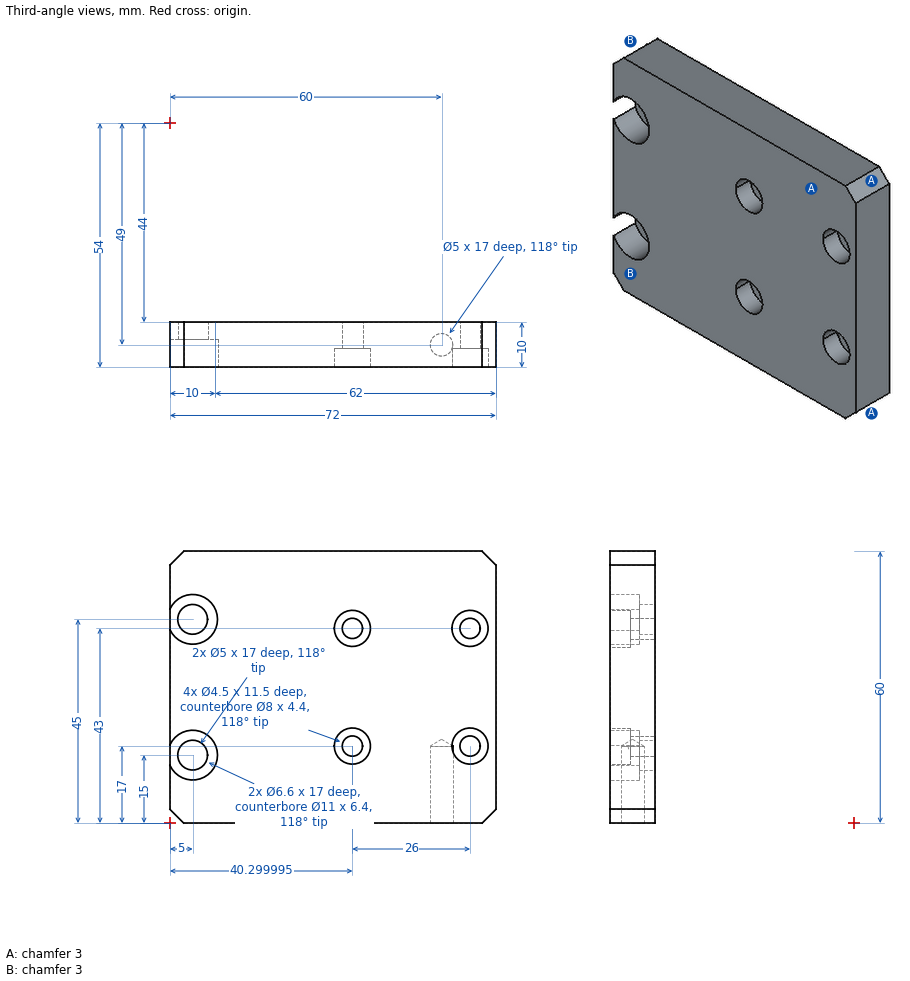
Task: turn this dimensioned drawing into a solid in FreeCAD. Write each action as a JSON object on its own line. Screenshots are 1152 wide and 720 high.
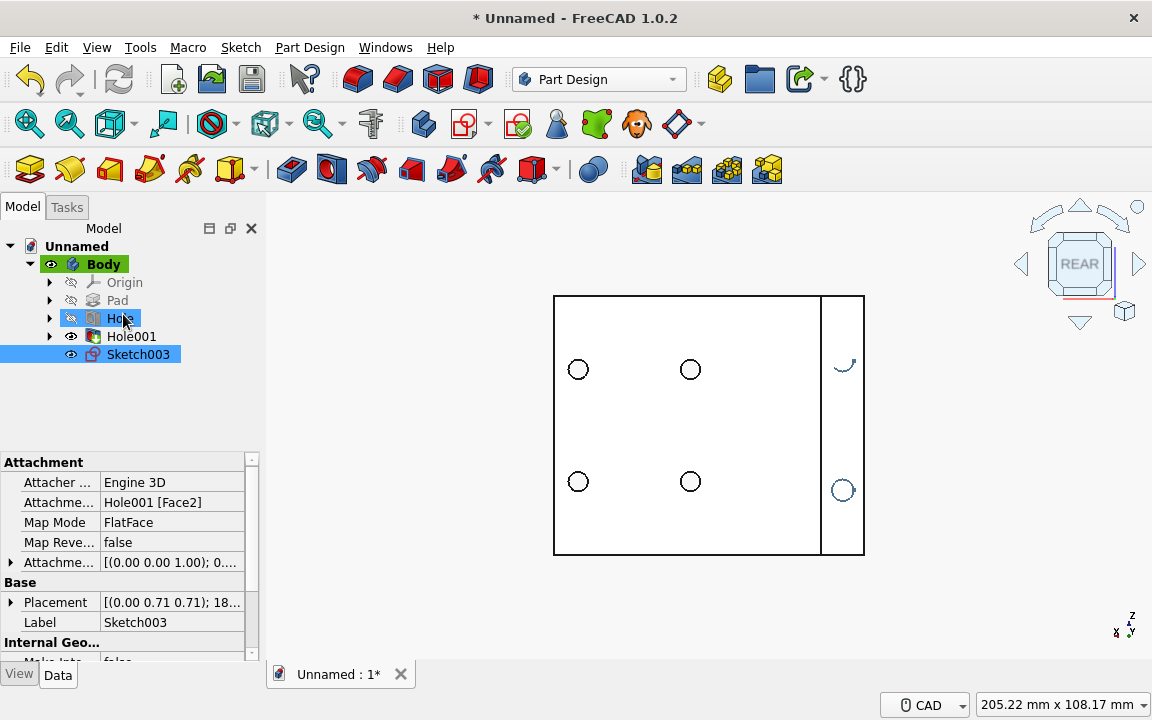
{"action": "left_click", "coordinate": [332, 170]}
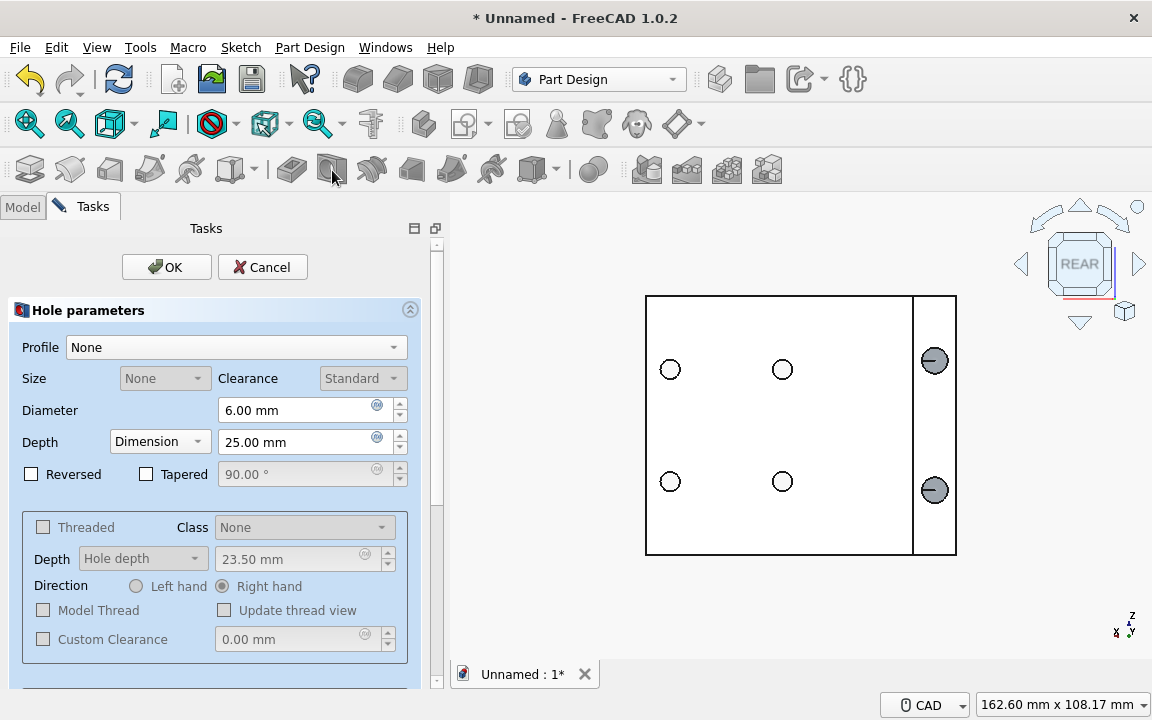
{"action": "triple_click", "coordinate": [305, 410]}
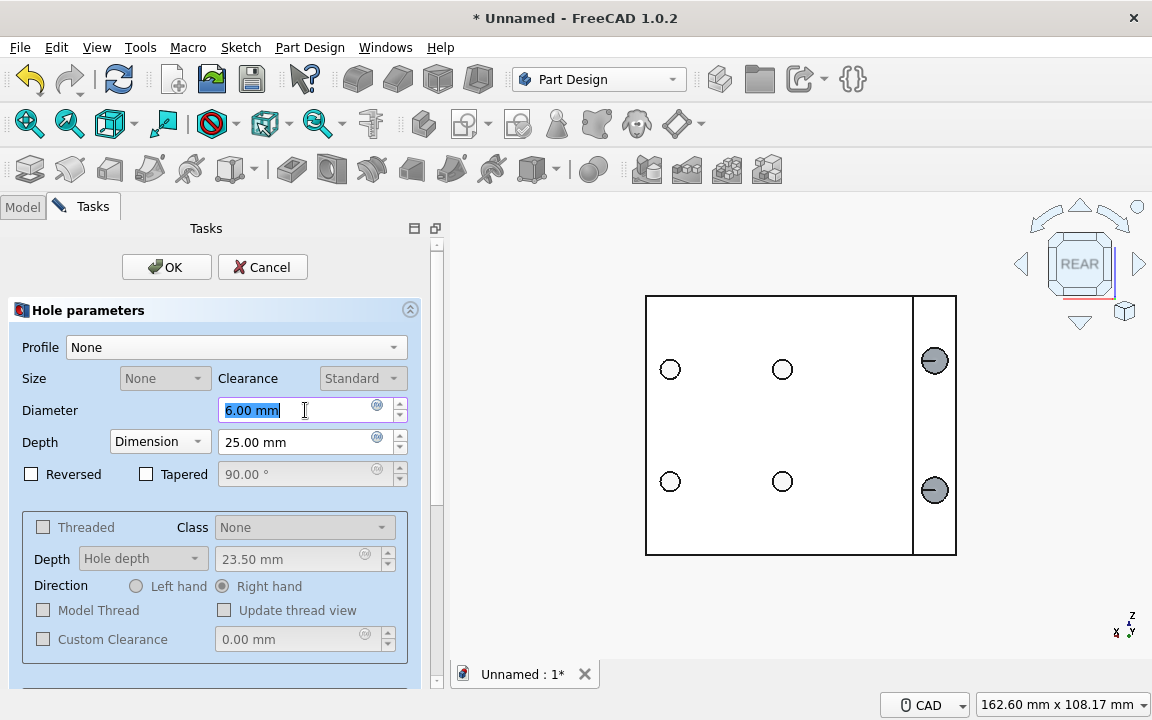
{"action": "type", "text": "5"}
{"action": "key", "text": "Tab"}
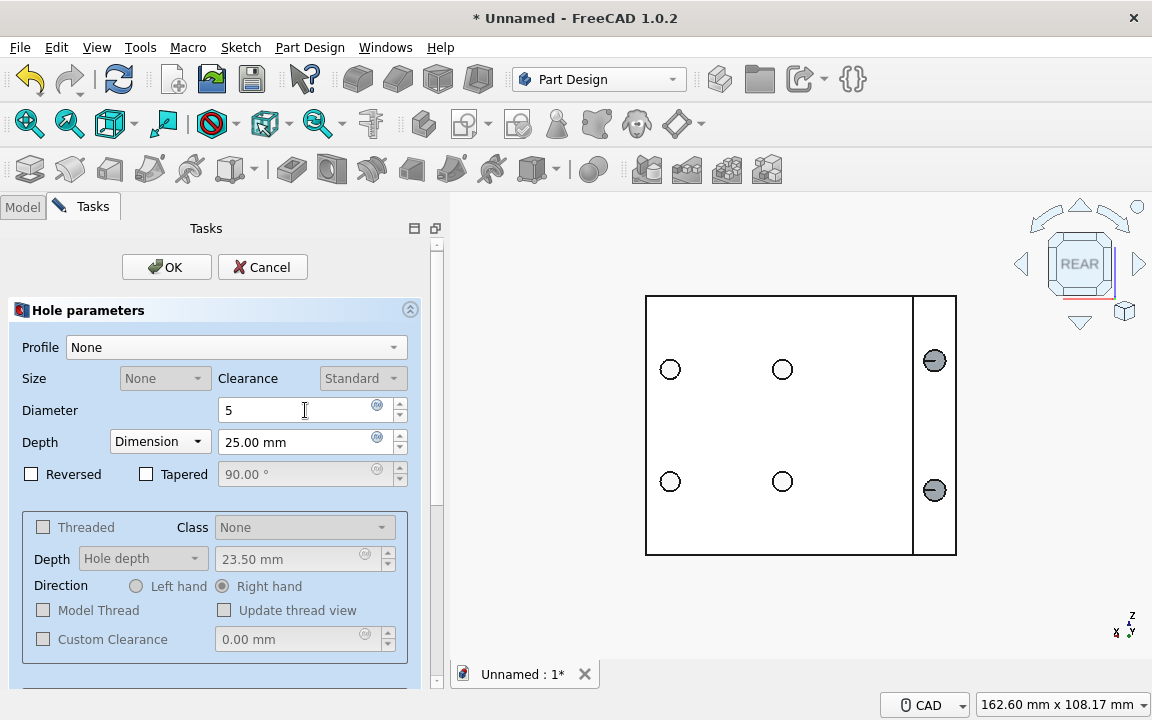
{"action": "triple_click", "coordinate": [305, 442]}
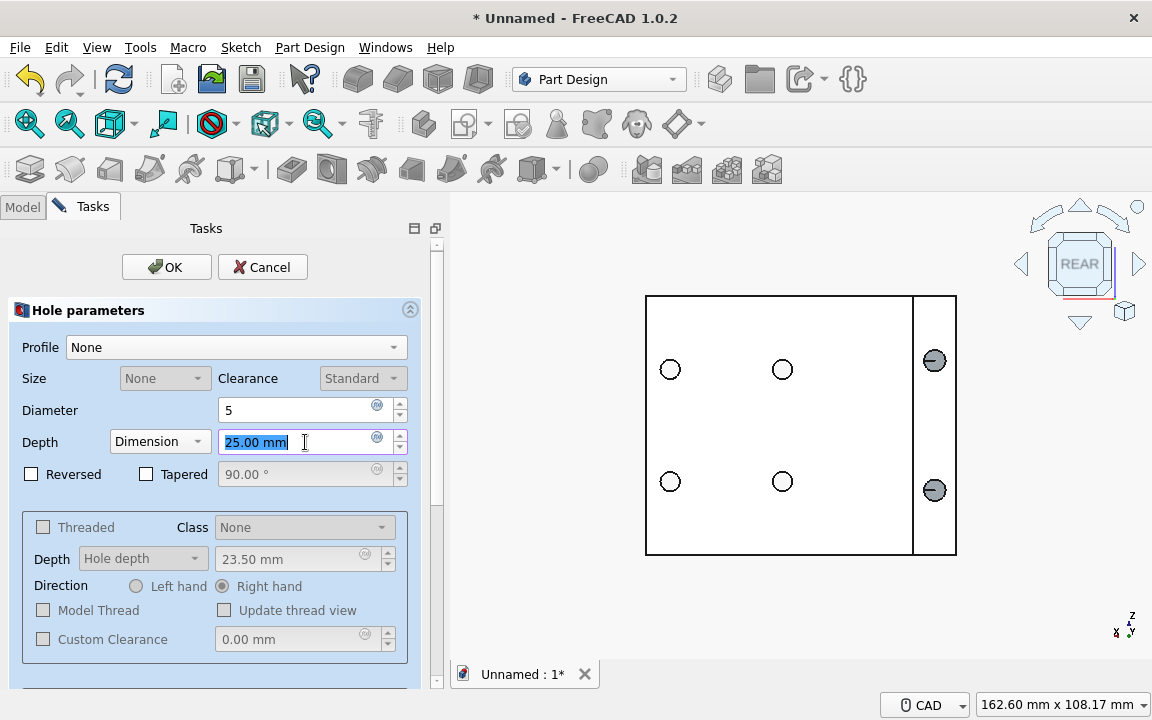
{"action": "type", "text": "17"}
{"action": "key", "text": "Tab"}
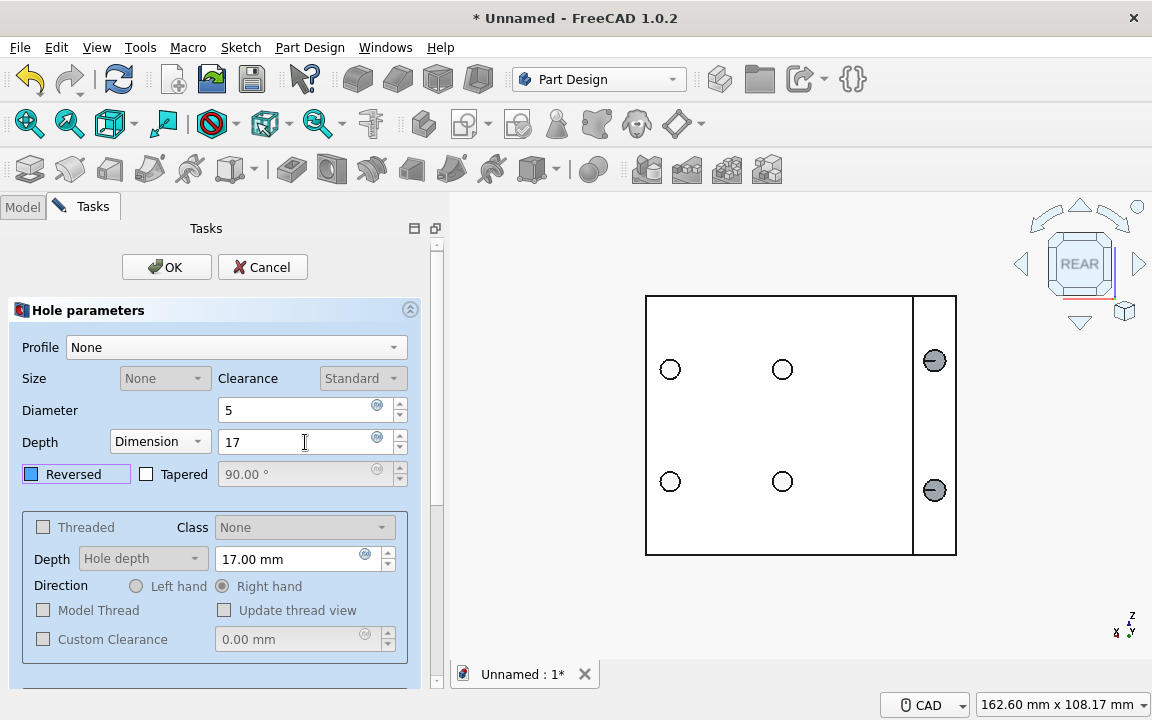
{"action": "left_click", "coordinate": [167, 267]}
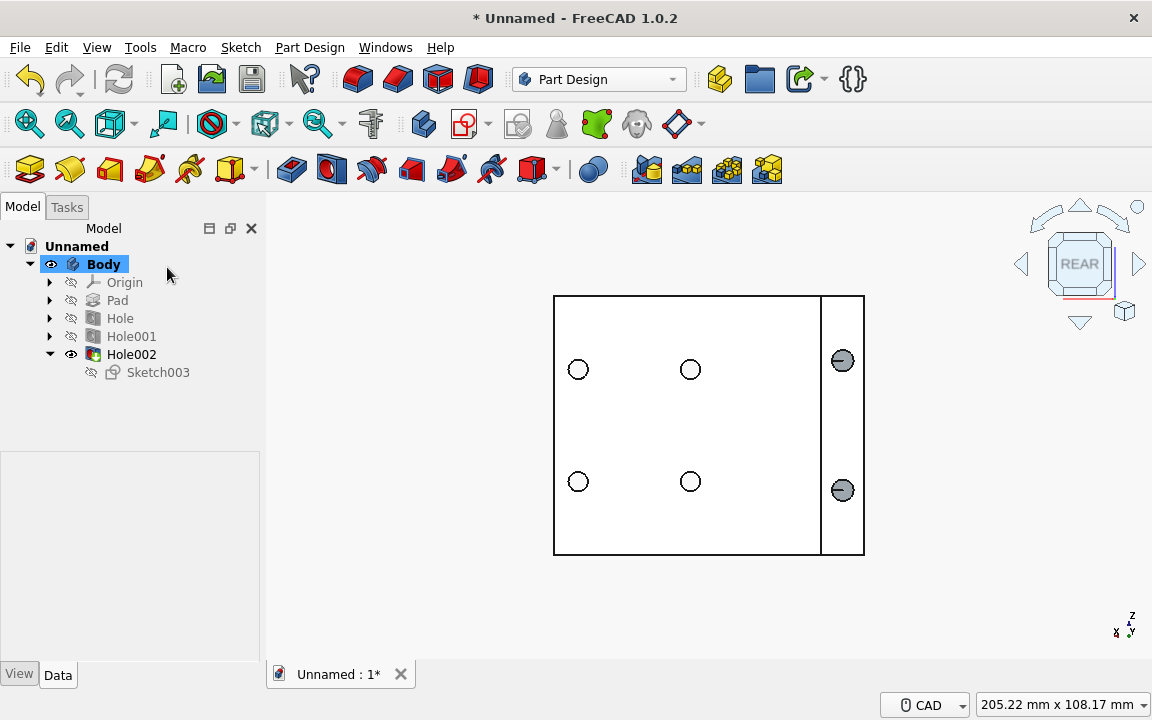
{"action": "left_click", "coordinate": [843, 295]}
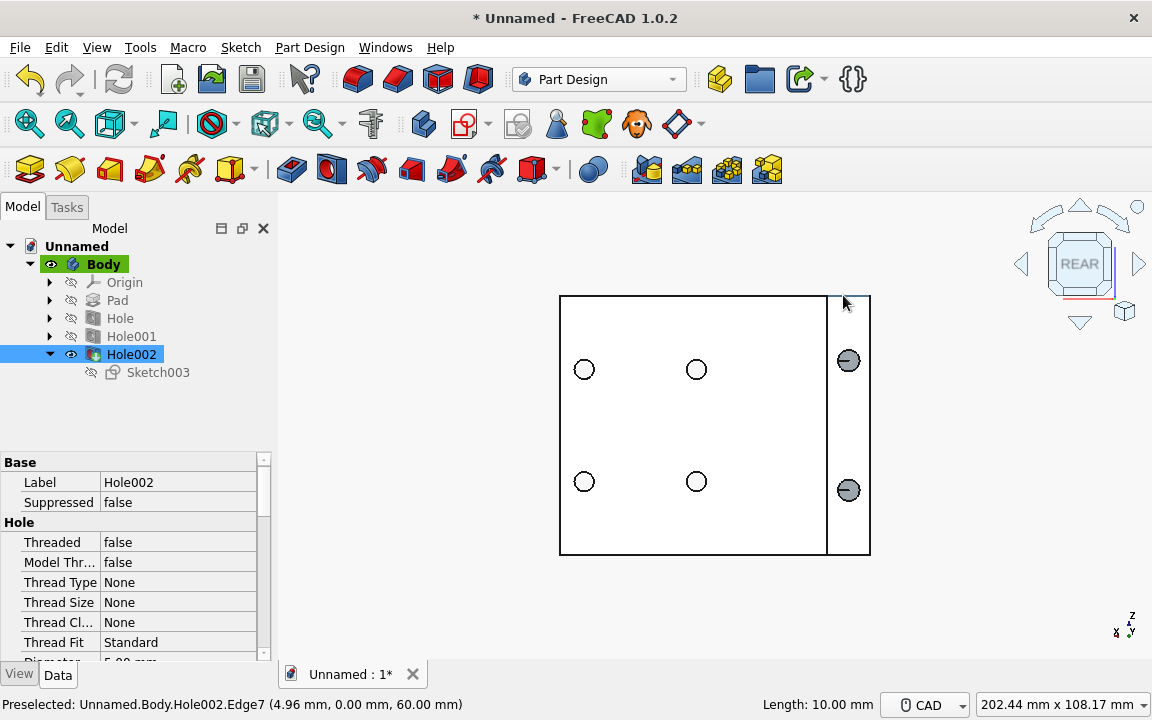
{"action": "key", "text": "0"}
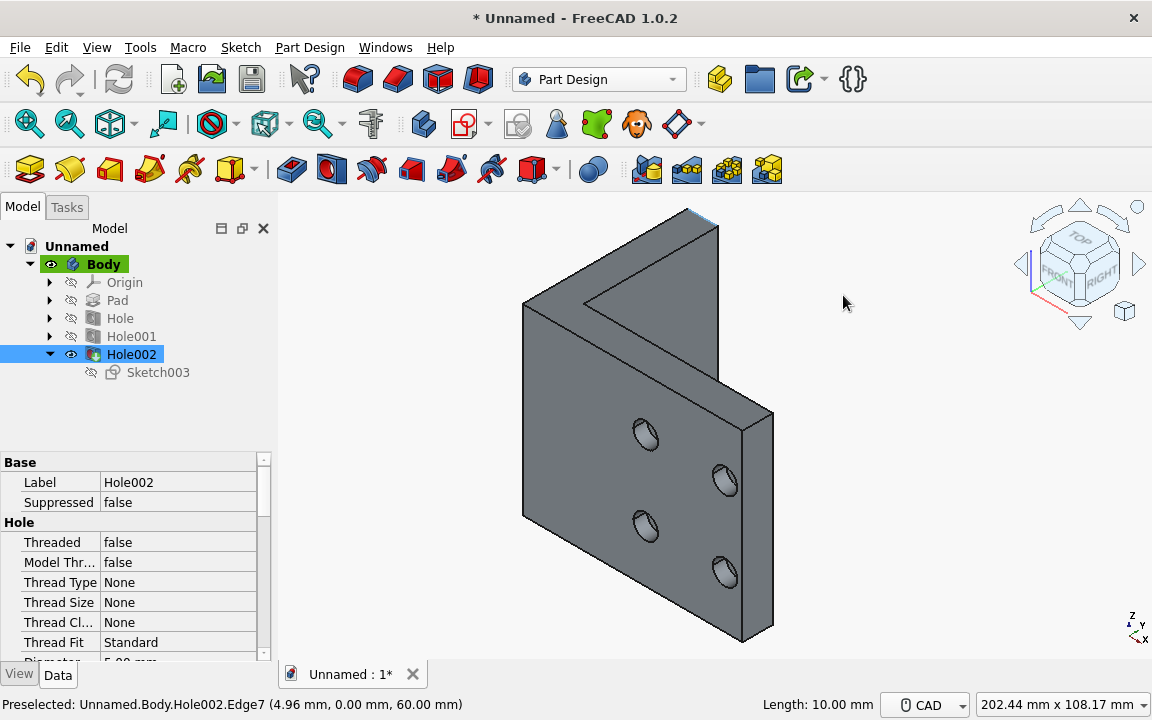
{"action": "left_click", "coordinate": [758, 421], "text": "ctrl"}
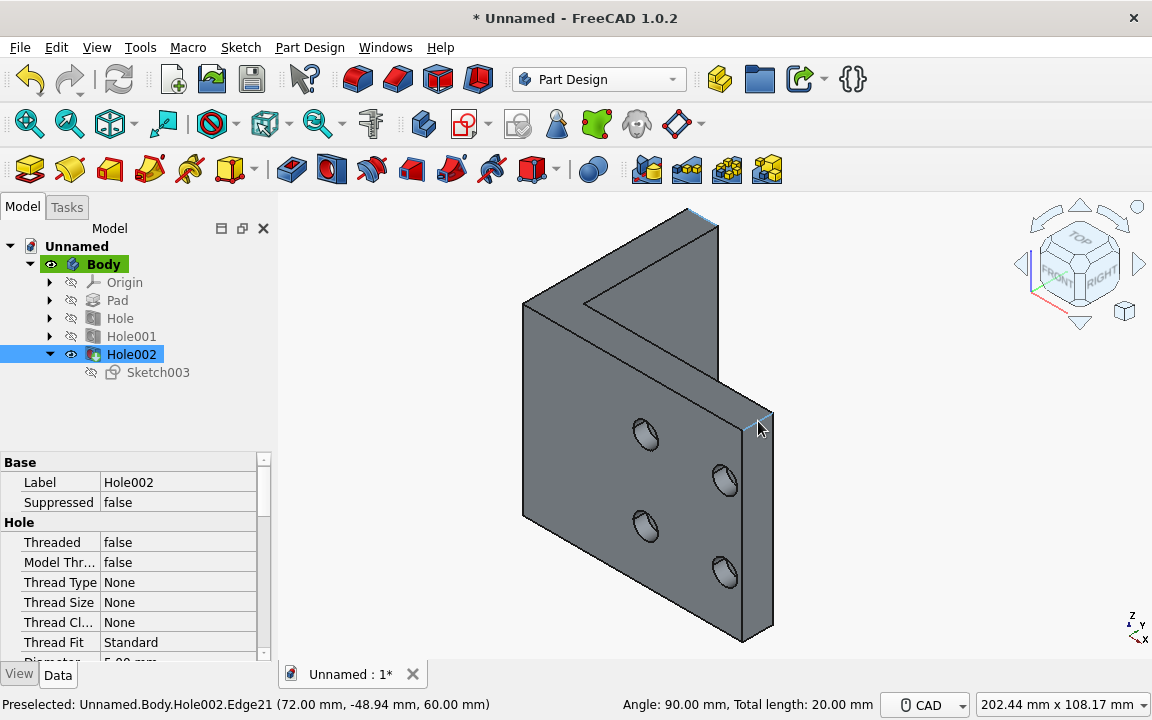
{"action": "key", "text": "2"}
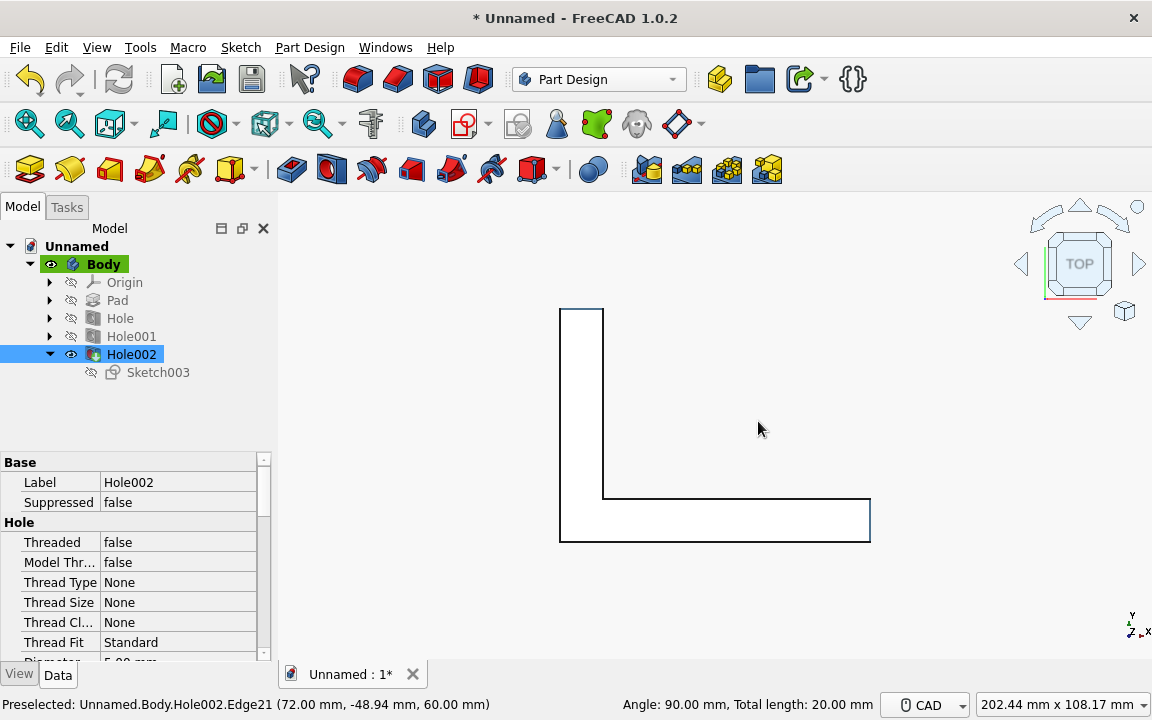
{"action": "key", "text": "1"}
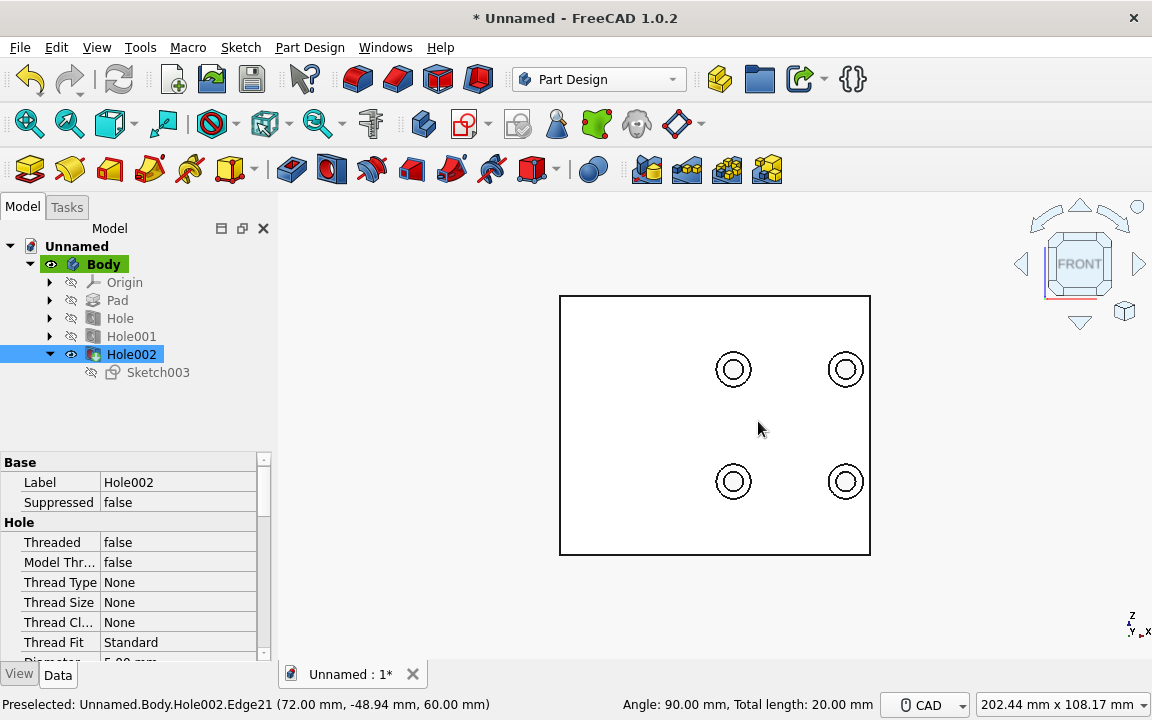
{"action": "key", "text": "3"}